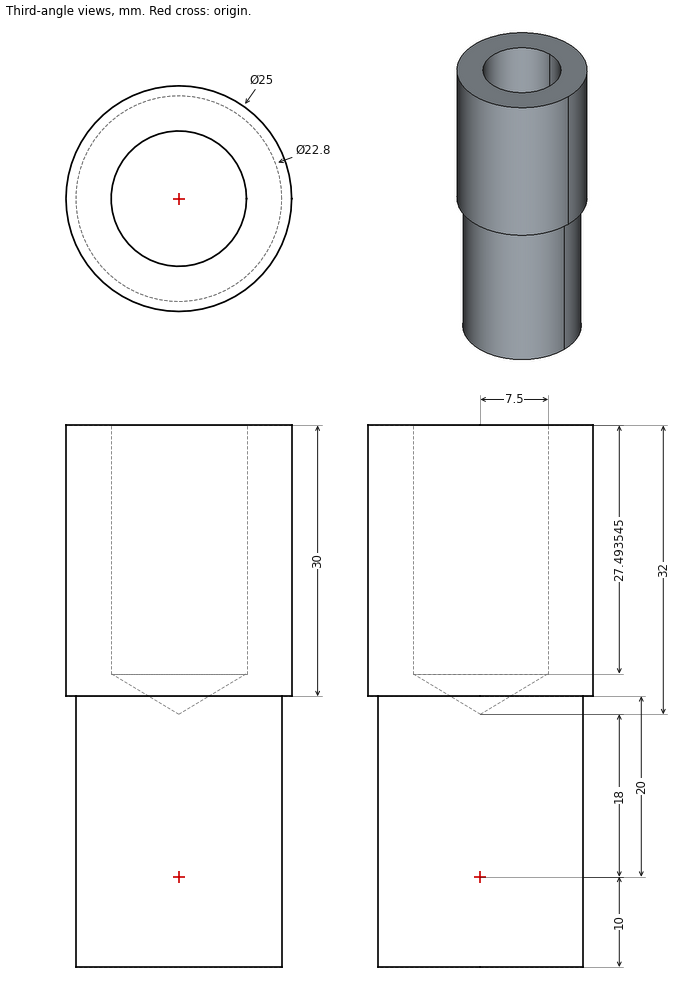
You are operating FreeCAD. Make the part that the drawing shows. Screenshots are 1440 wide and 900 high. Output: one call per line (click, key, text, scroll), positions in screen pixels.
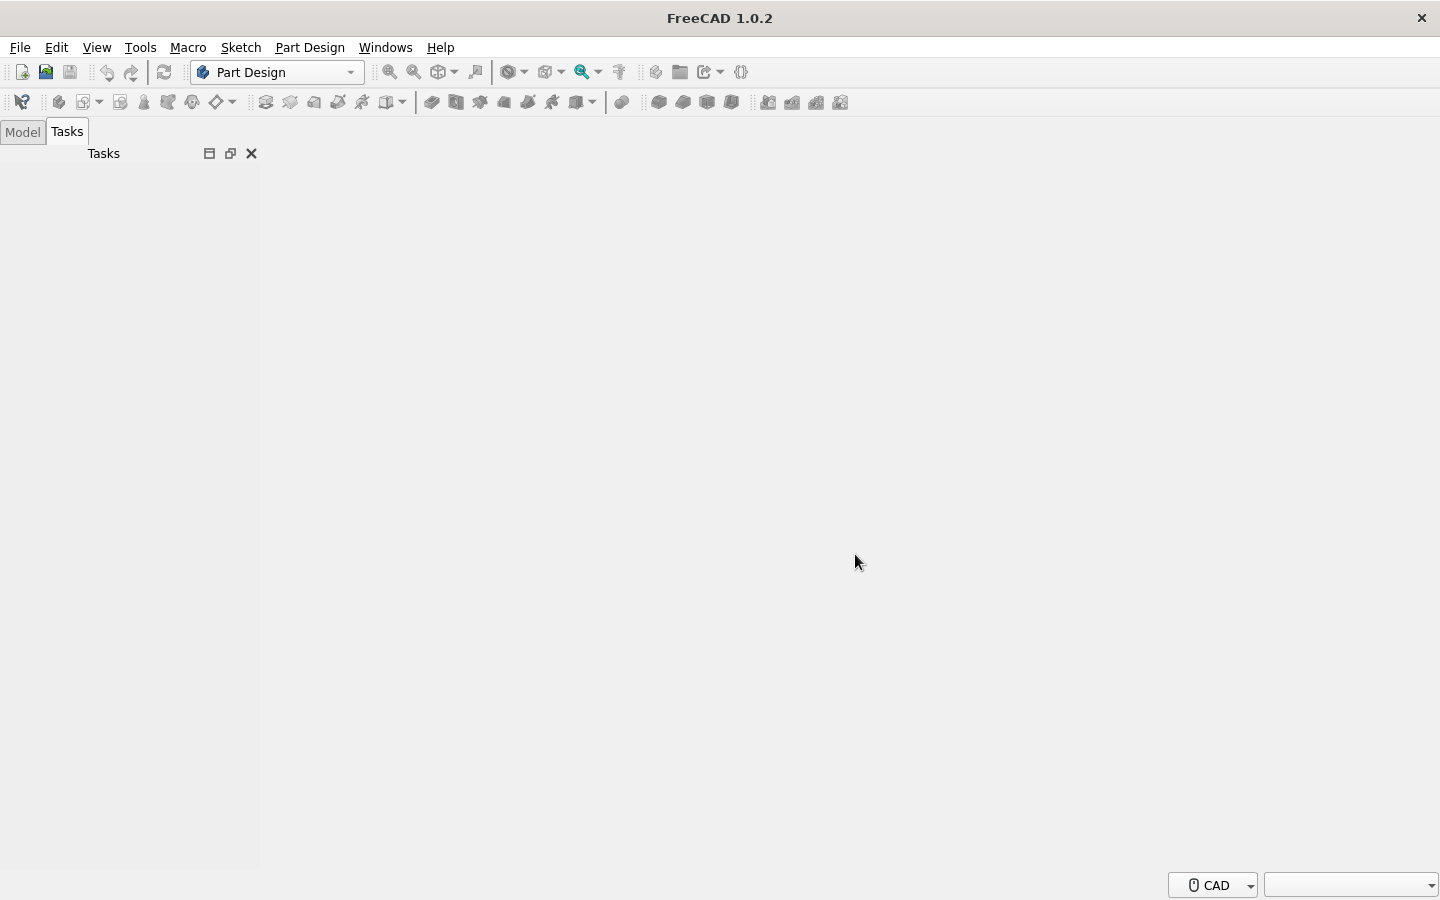
click(22, 72)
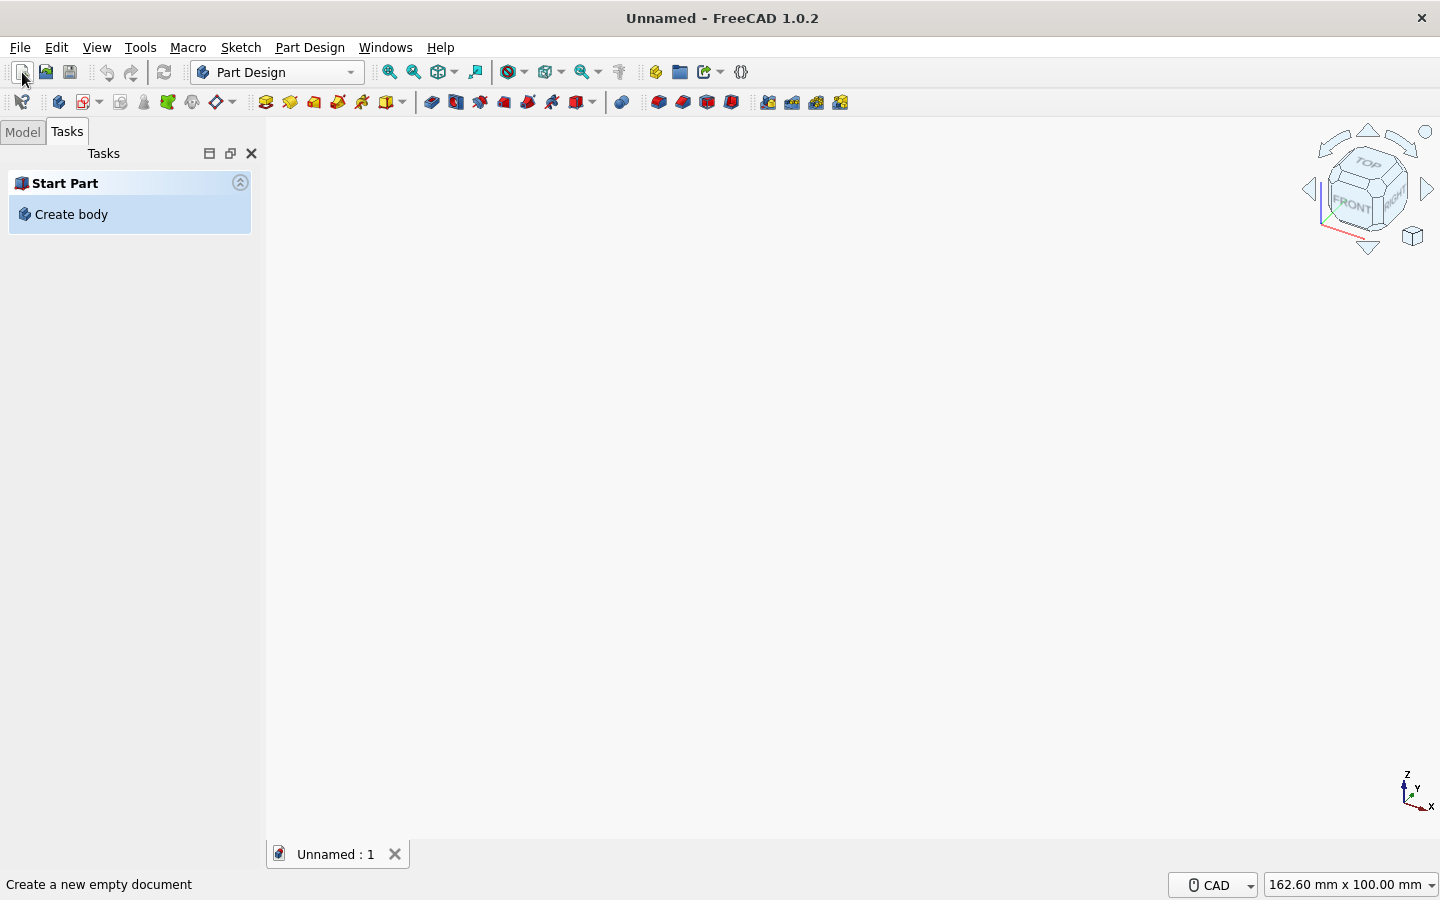
click(84, 102)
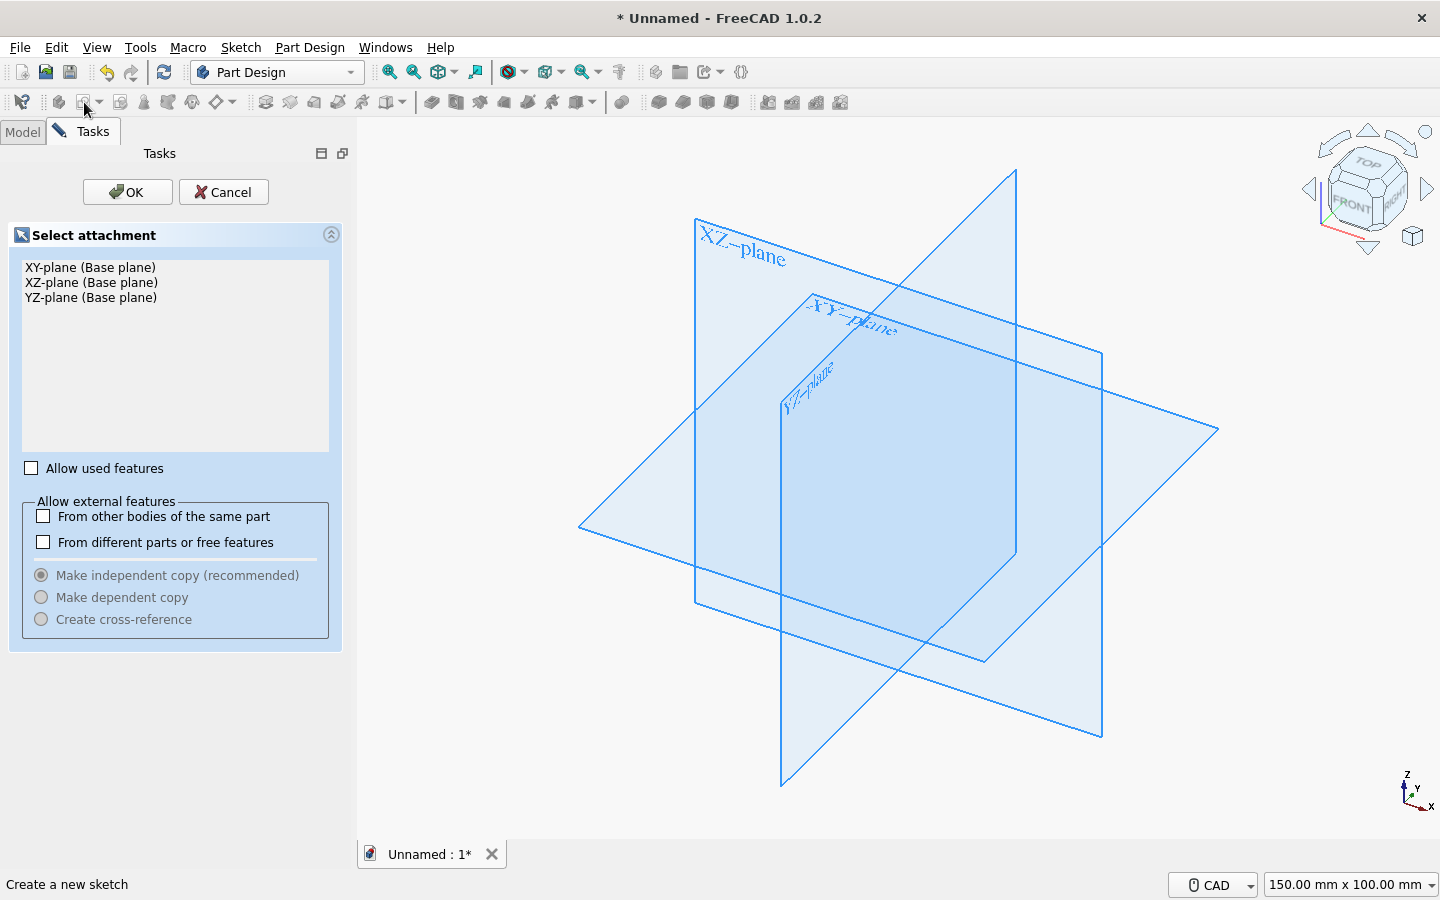
click(82, 268)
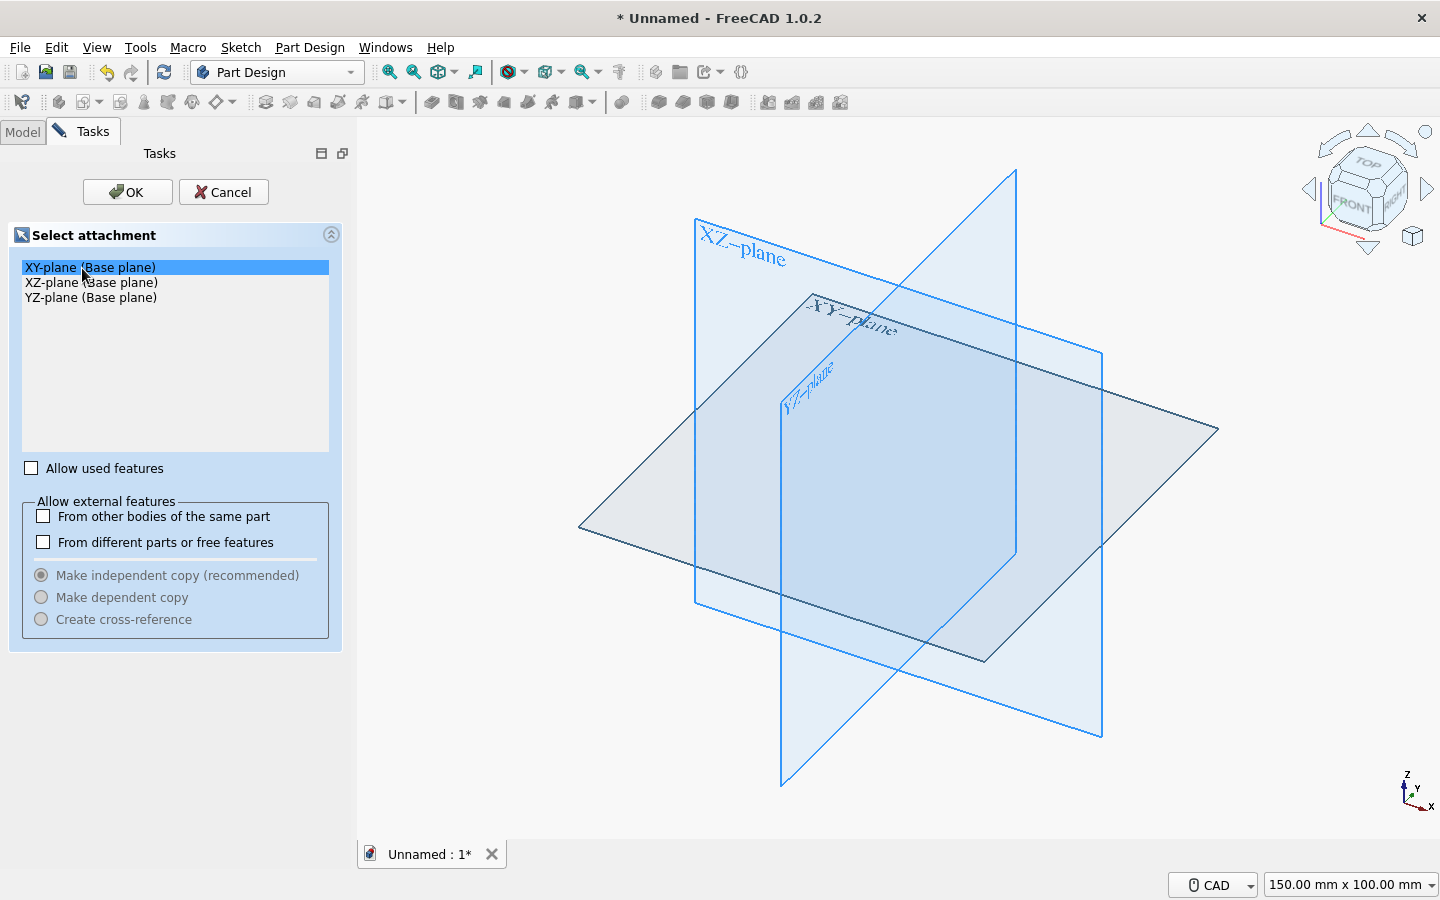
click(128, 192)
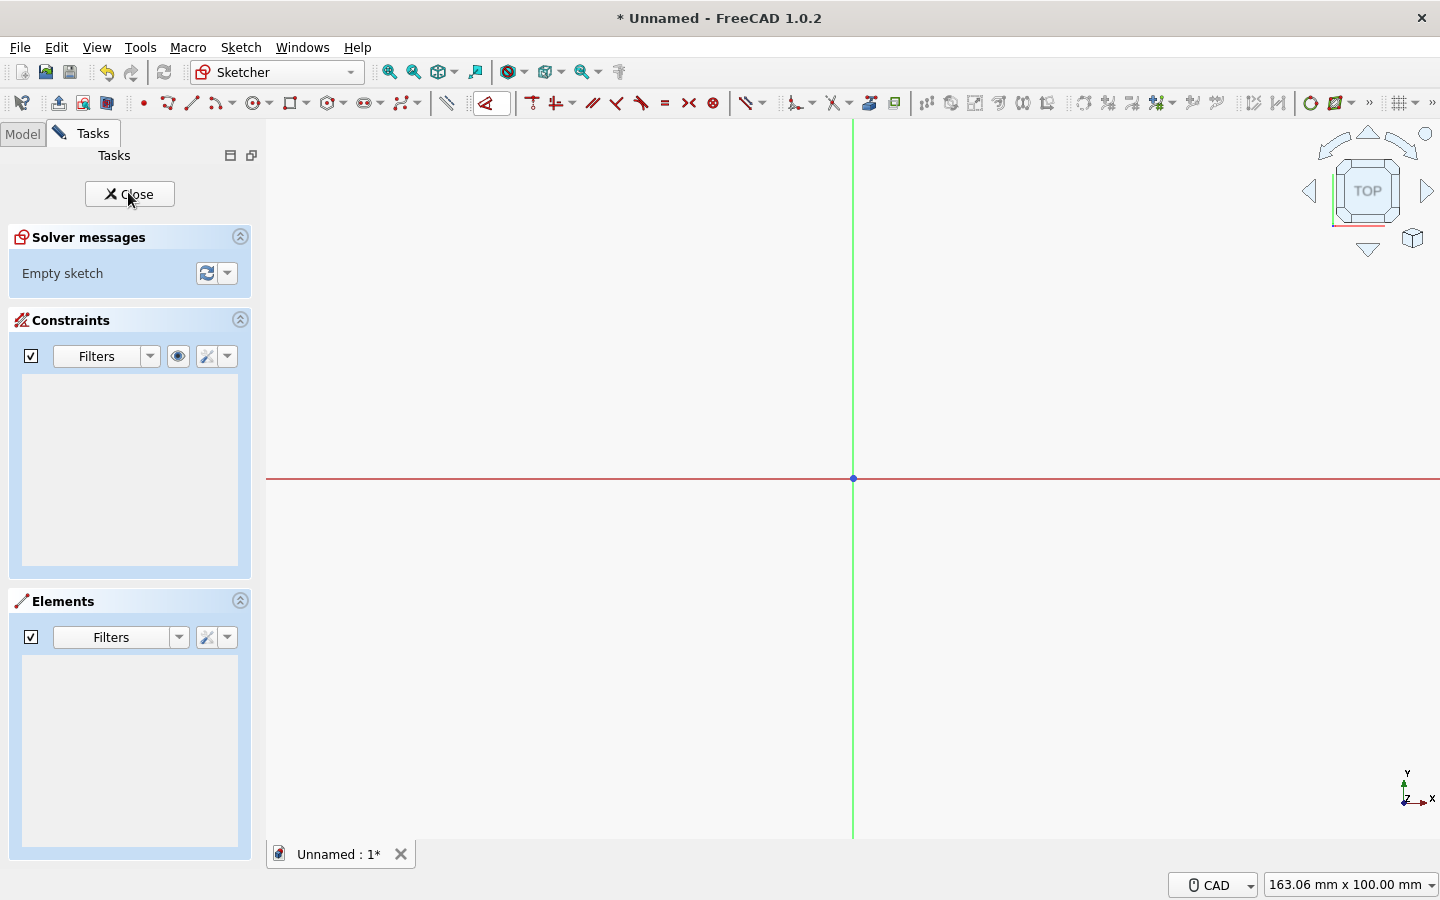
scroll(893, 479, up, 5)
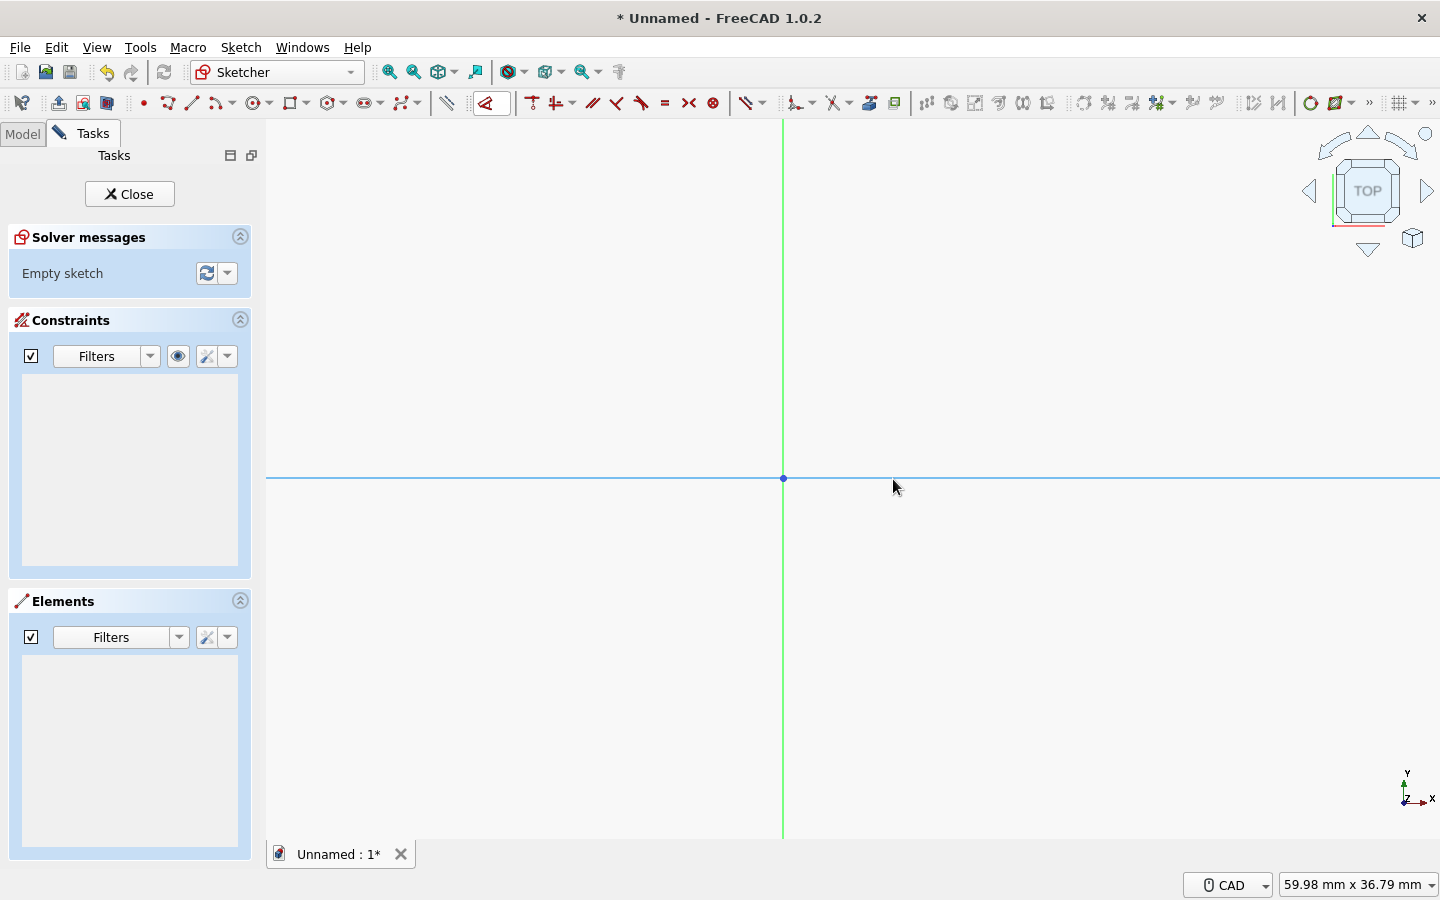
click(254, 104)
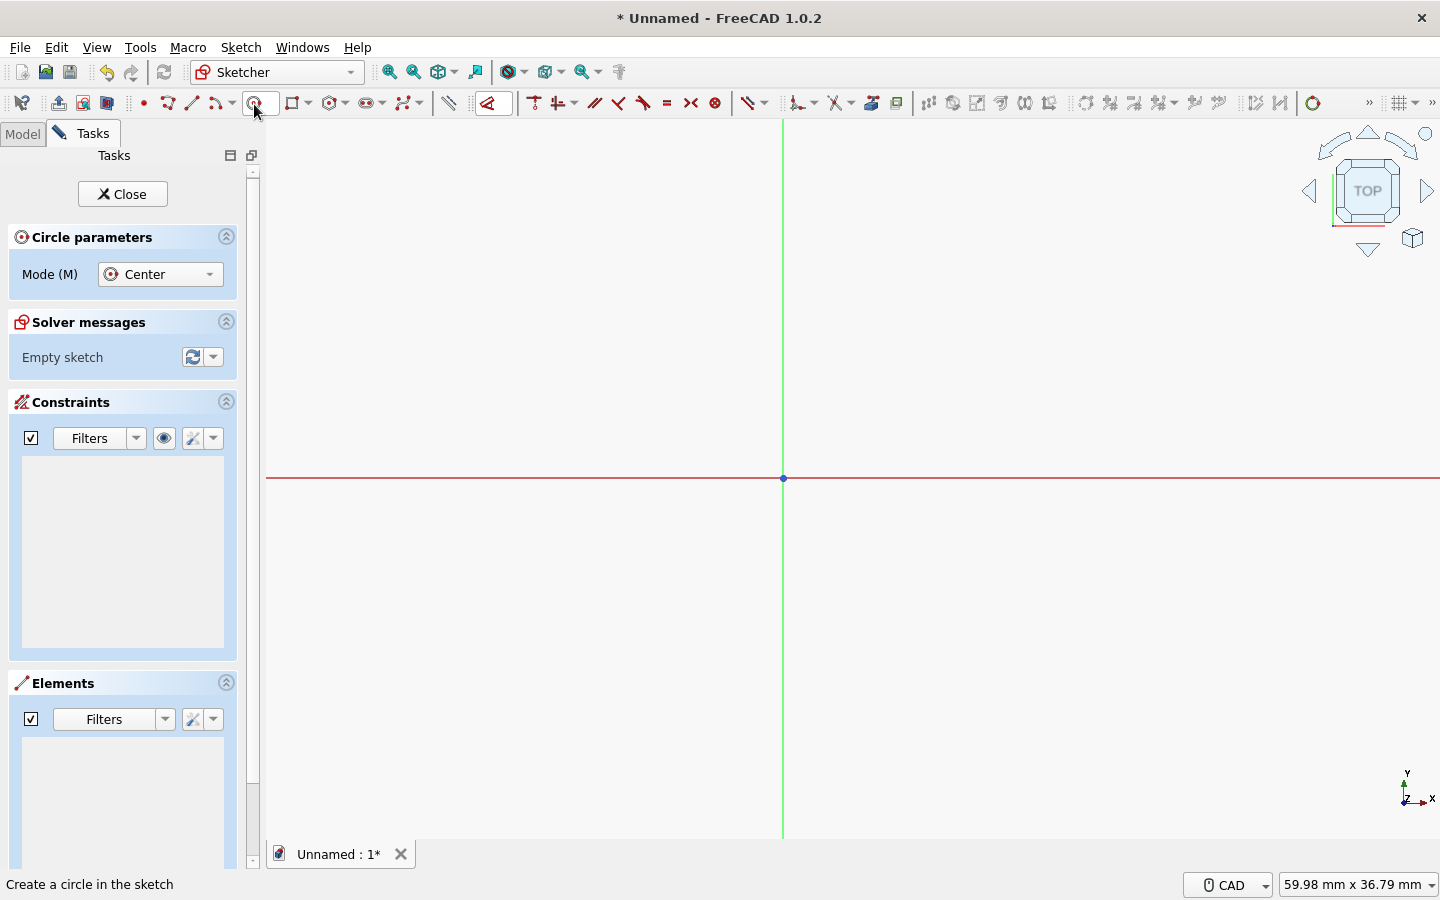
click(783, 478)
move(941, 320)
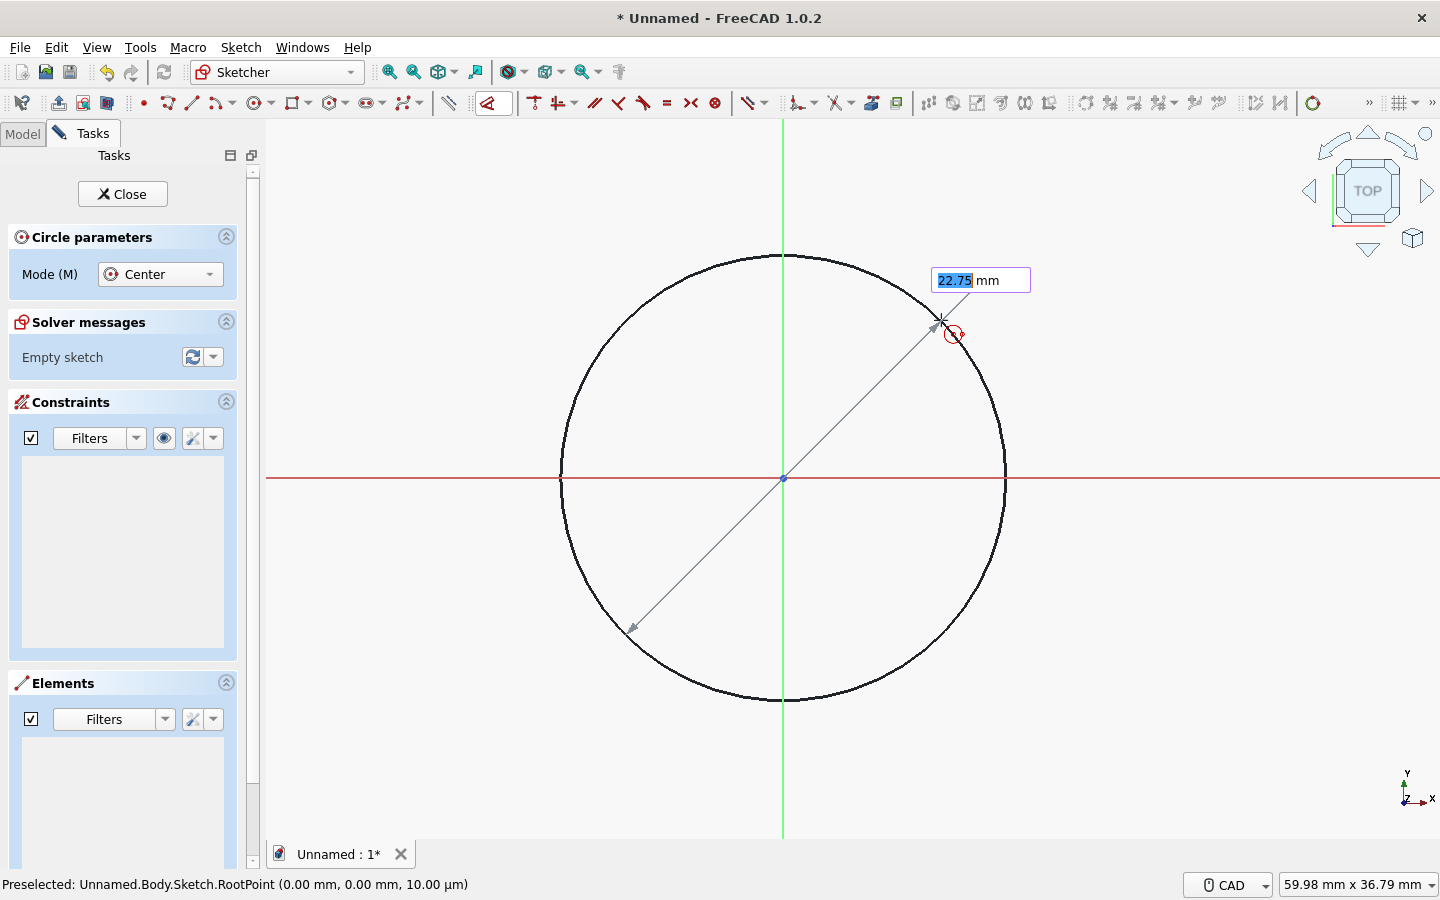
text(22.8)
key(Return)
key(Escape)